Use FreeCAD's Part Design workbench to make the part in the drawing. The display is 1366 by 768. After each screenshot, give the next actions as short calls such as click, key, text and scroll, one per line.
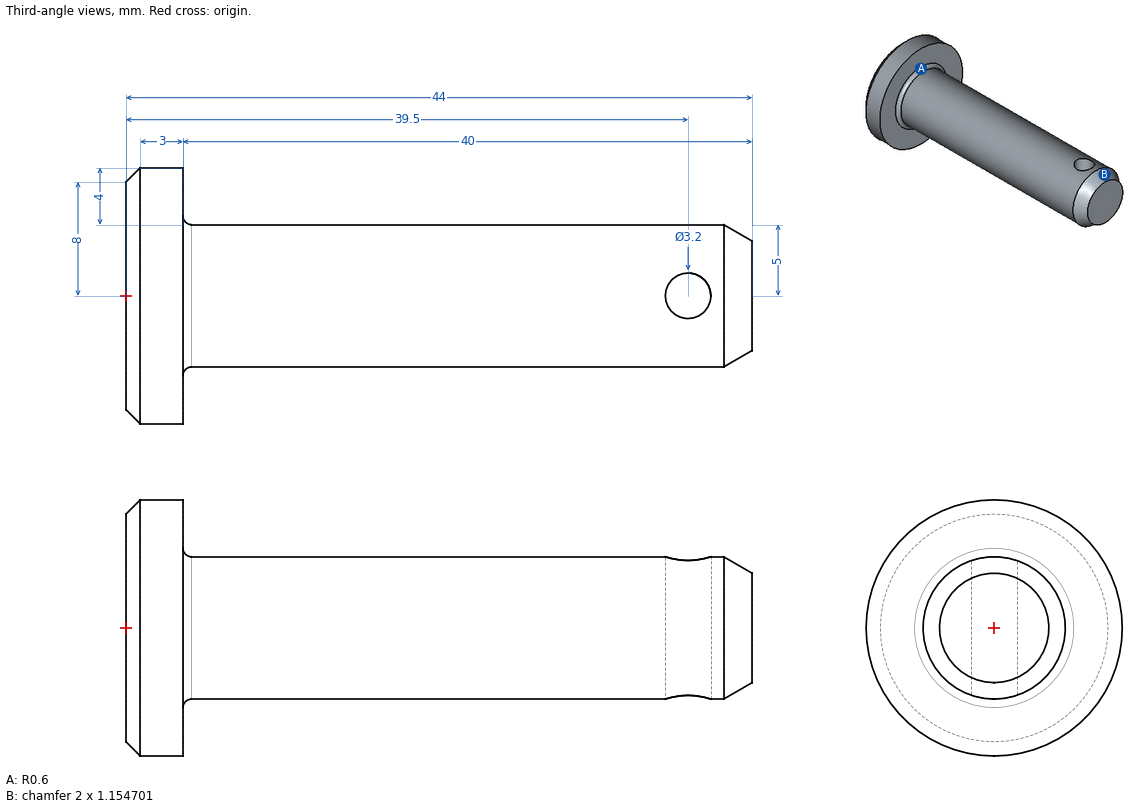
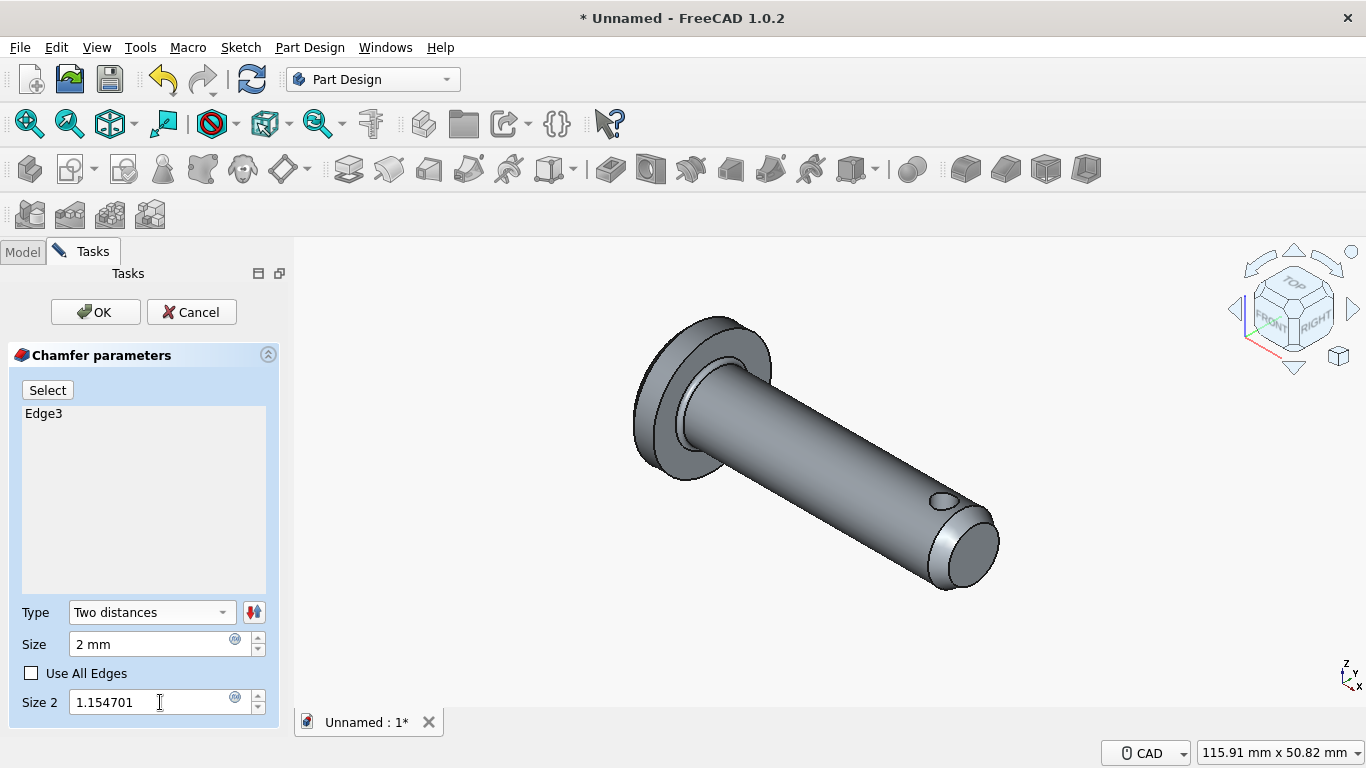
click(96, 312)